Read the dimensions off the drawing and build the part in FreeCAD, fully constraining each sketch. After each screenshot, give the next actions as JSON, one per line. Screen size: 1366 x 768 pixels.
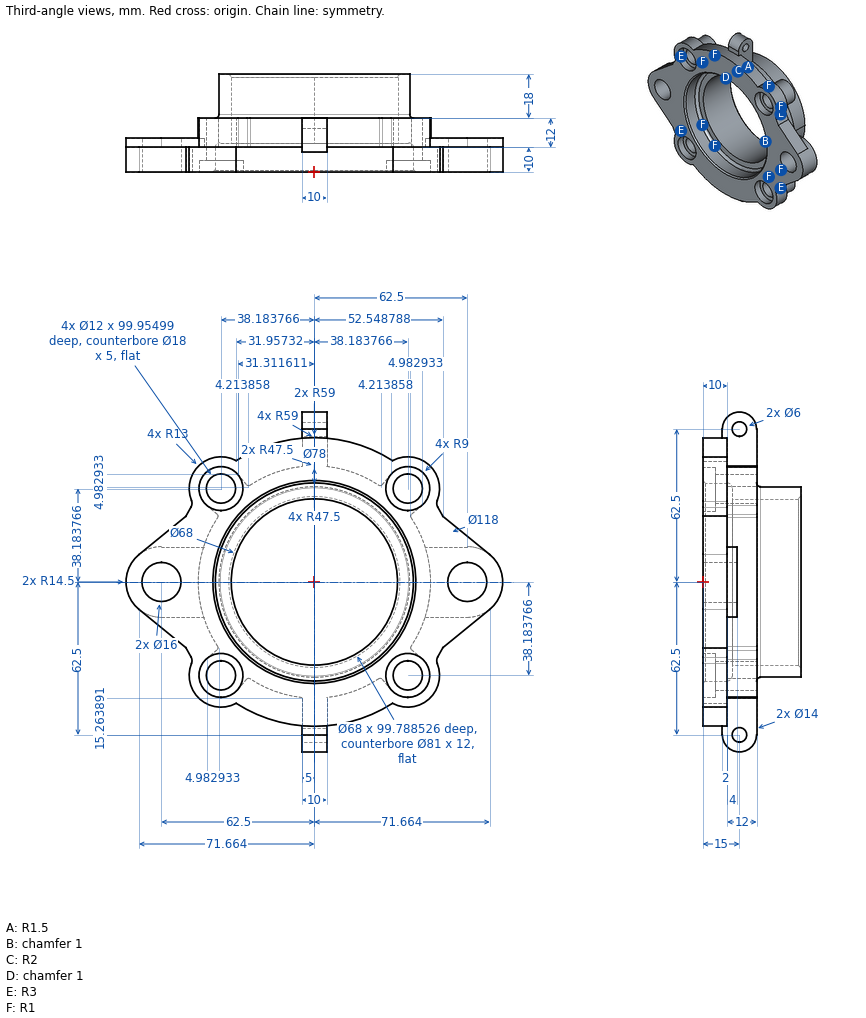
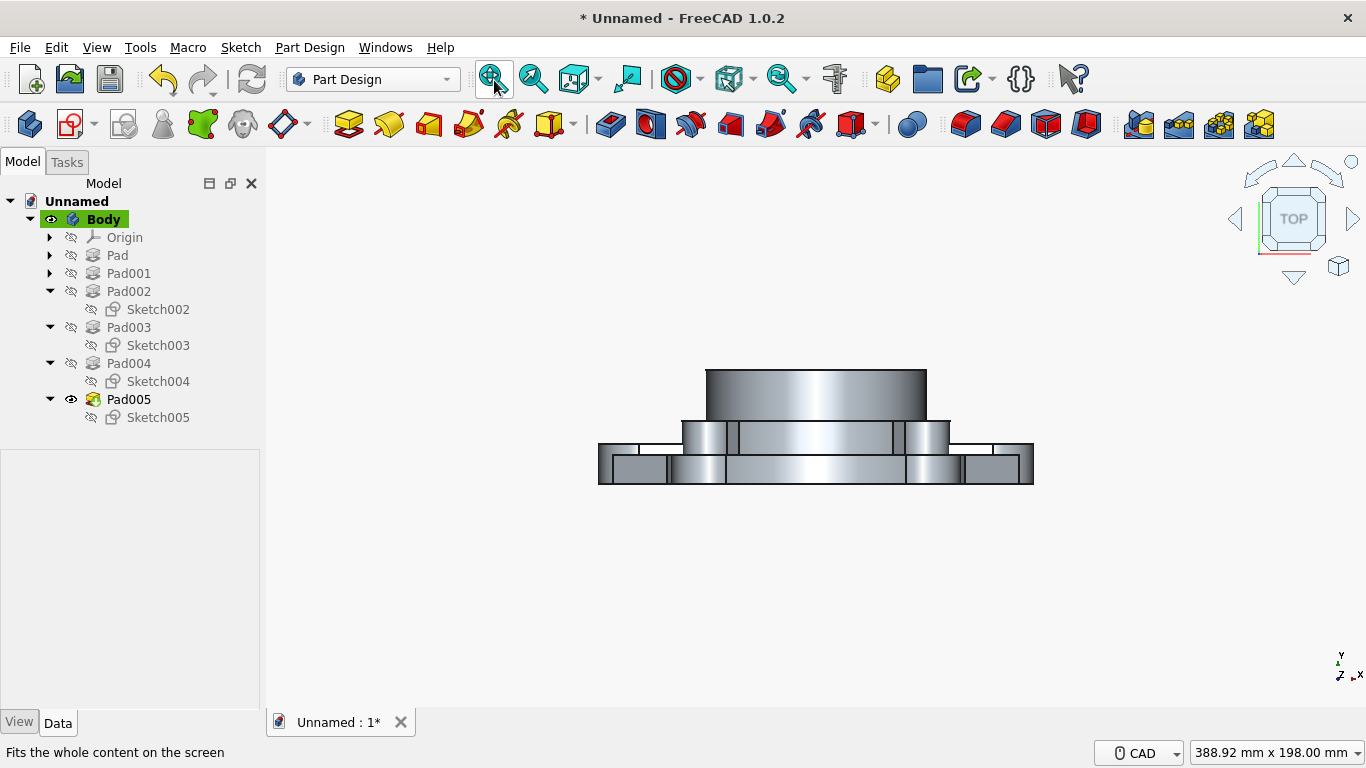
{"action": "left_click", "coordinate": [494, 80]}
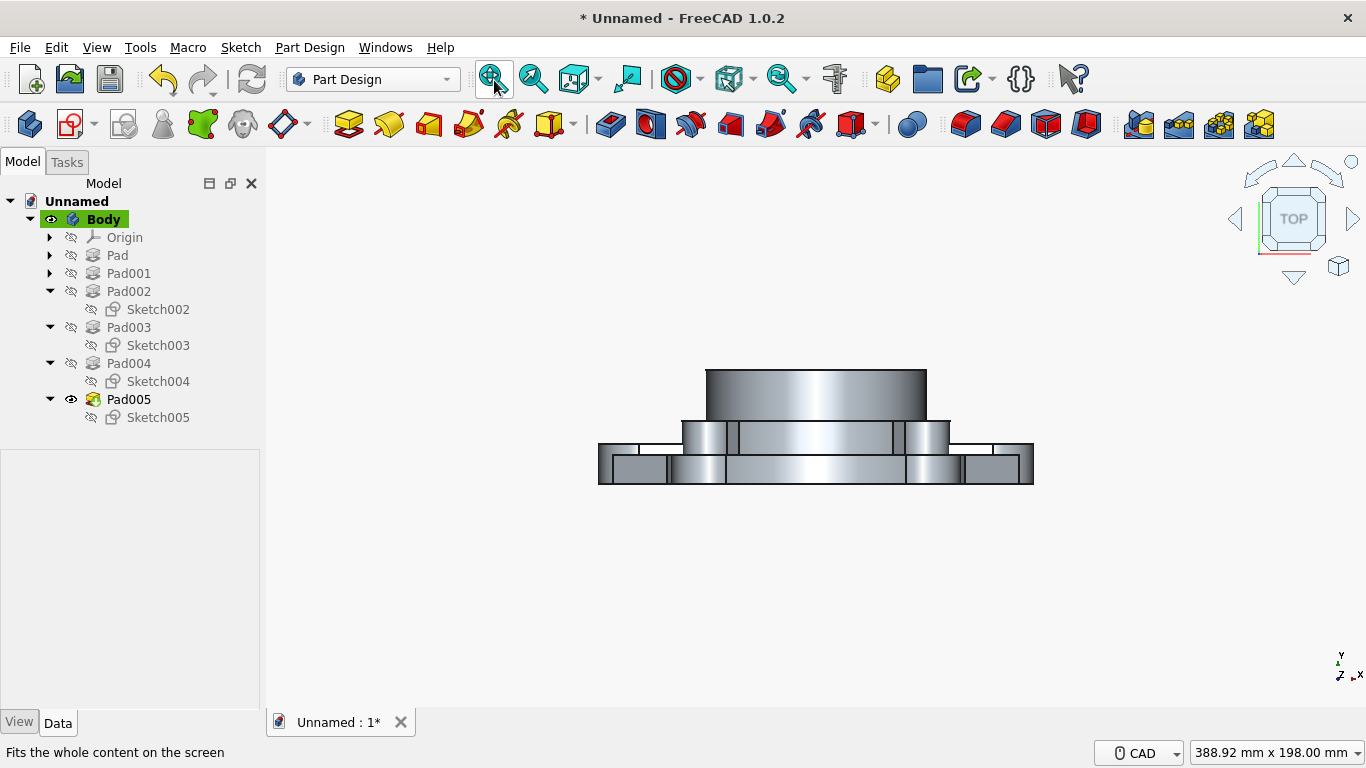
{"action": "key", "text": "1"}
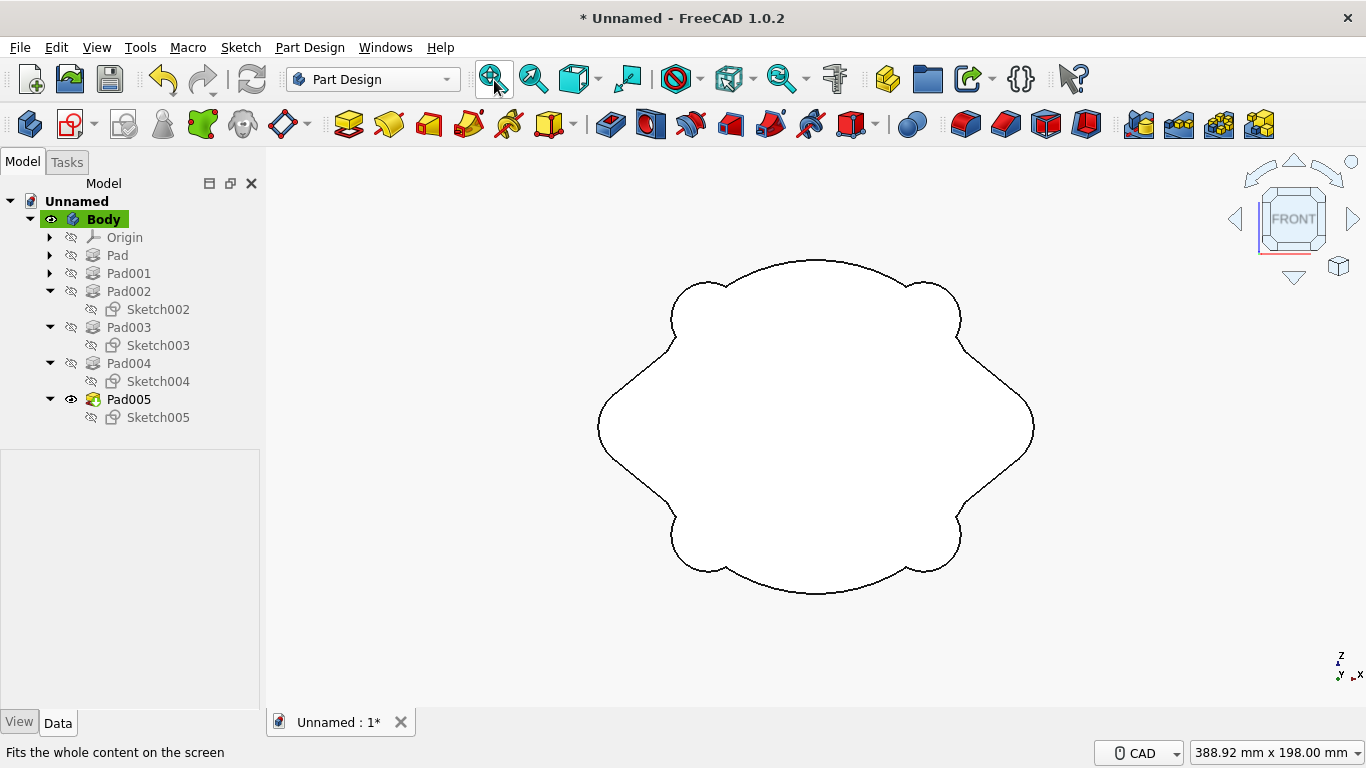
{"action": "key", "text": "3"}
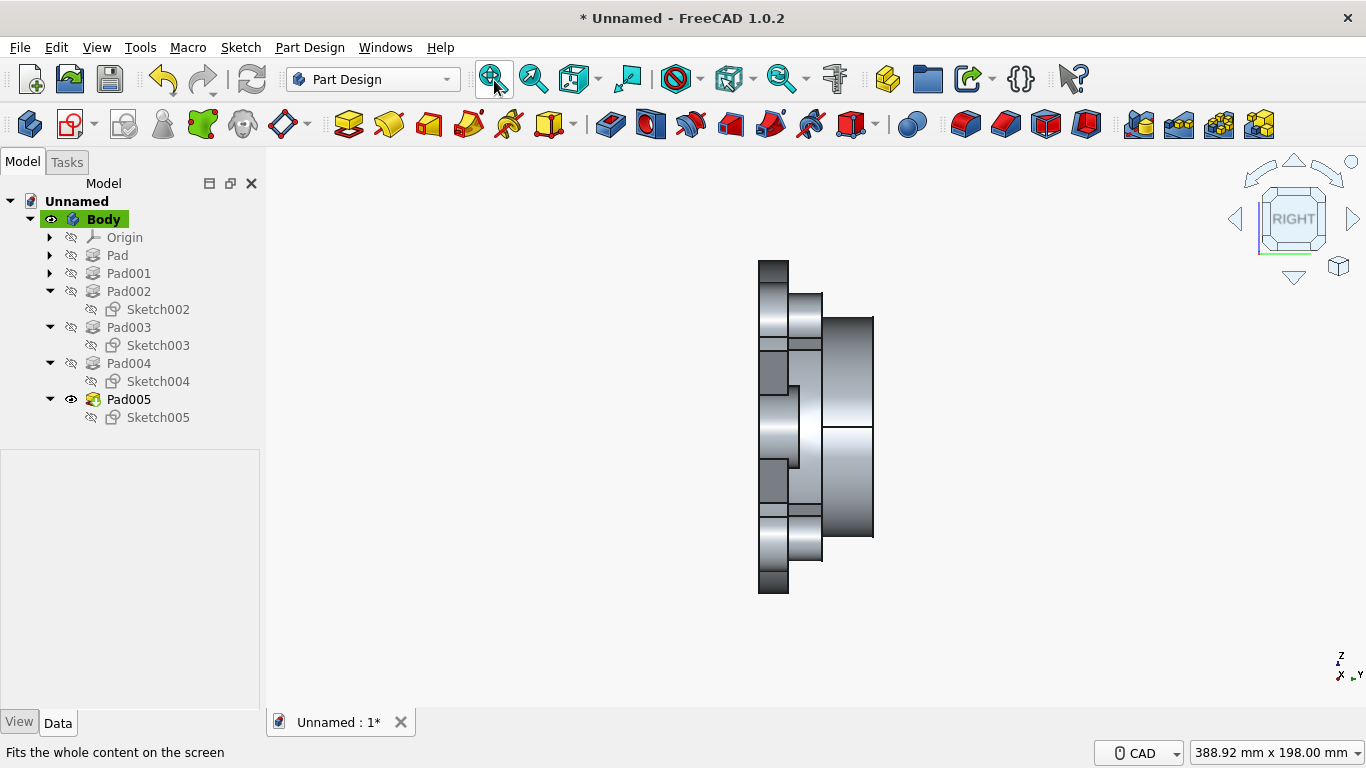
{"action": "key", "text": "5"}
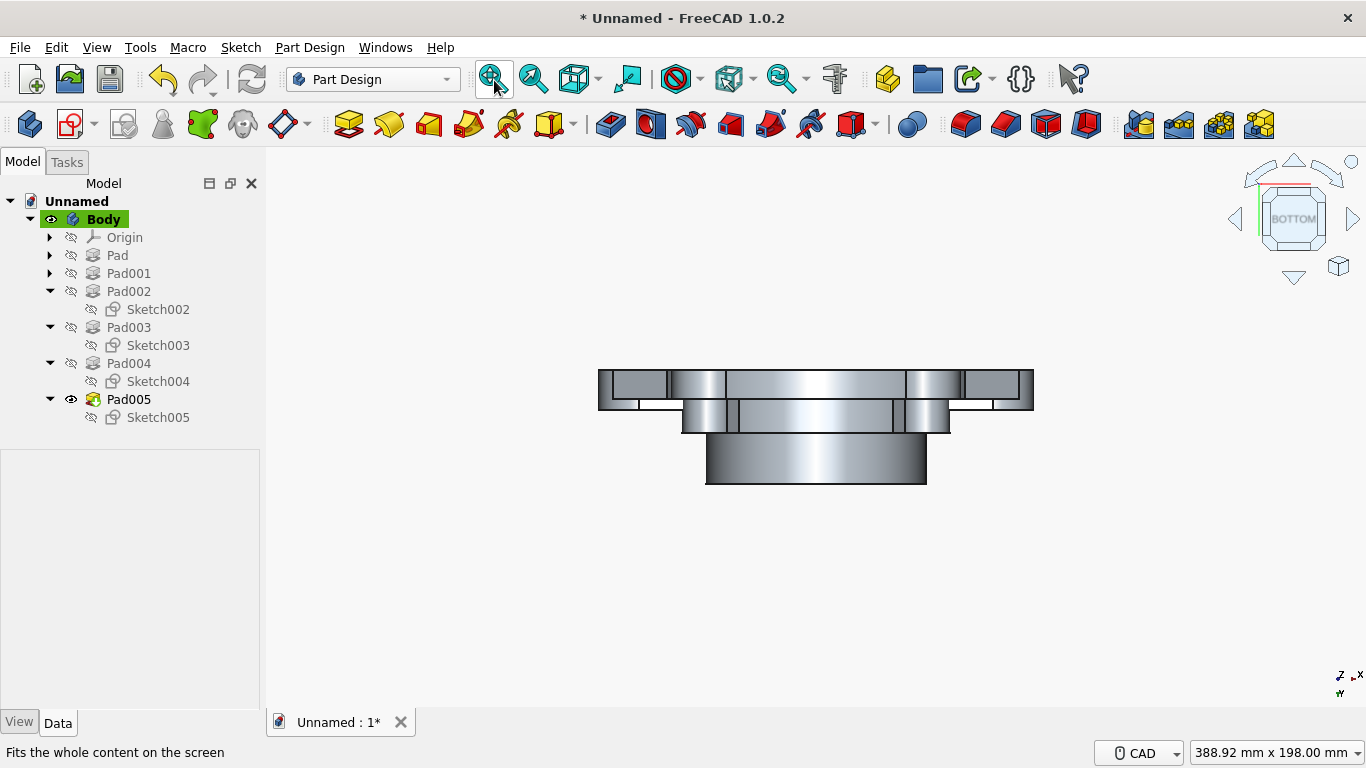
{"action": "left_click", "coordinate": [494, 80]}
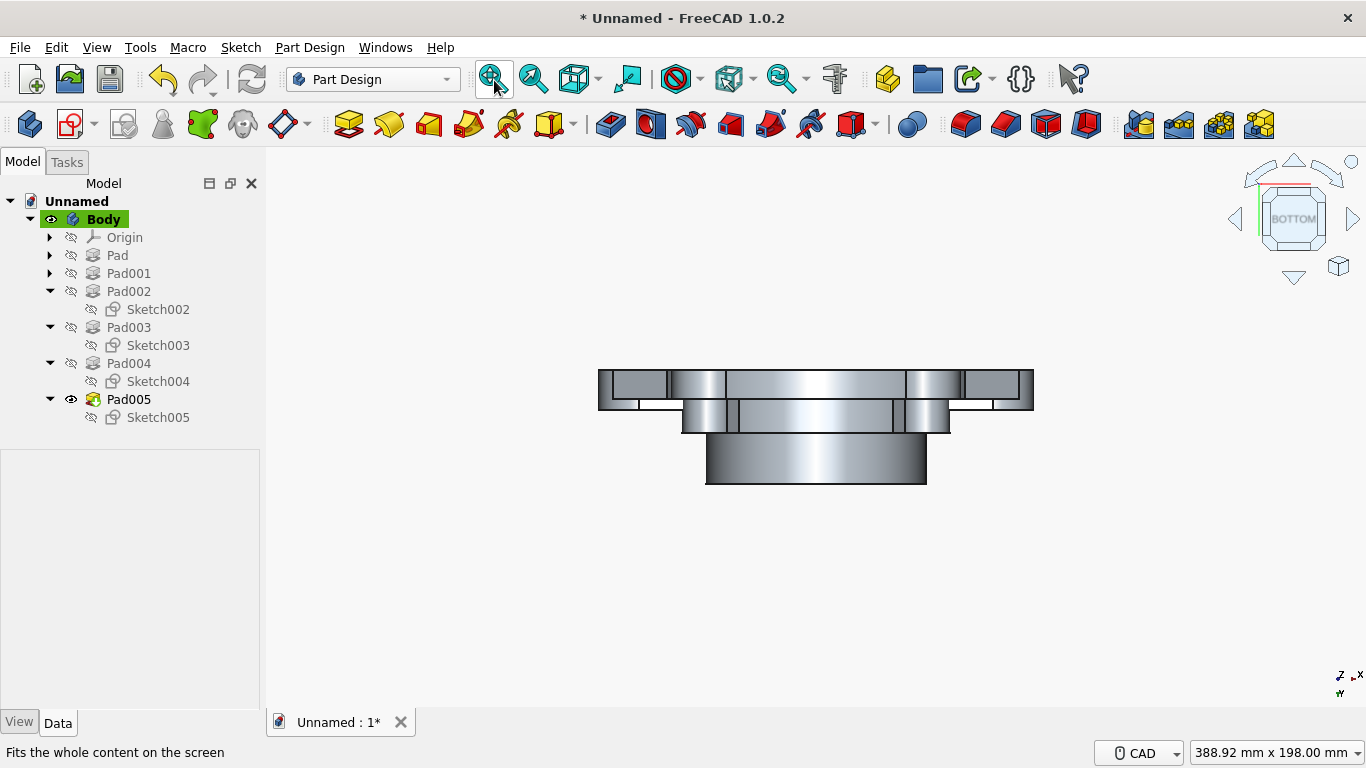
{"action": "key", "text": "4"}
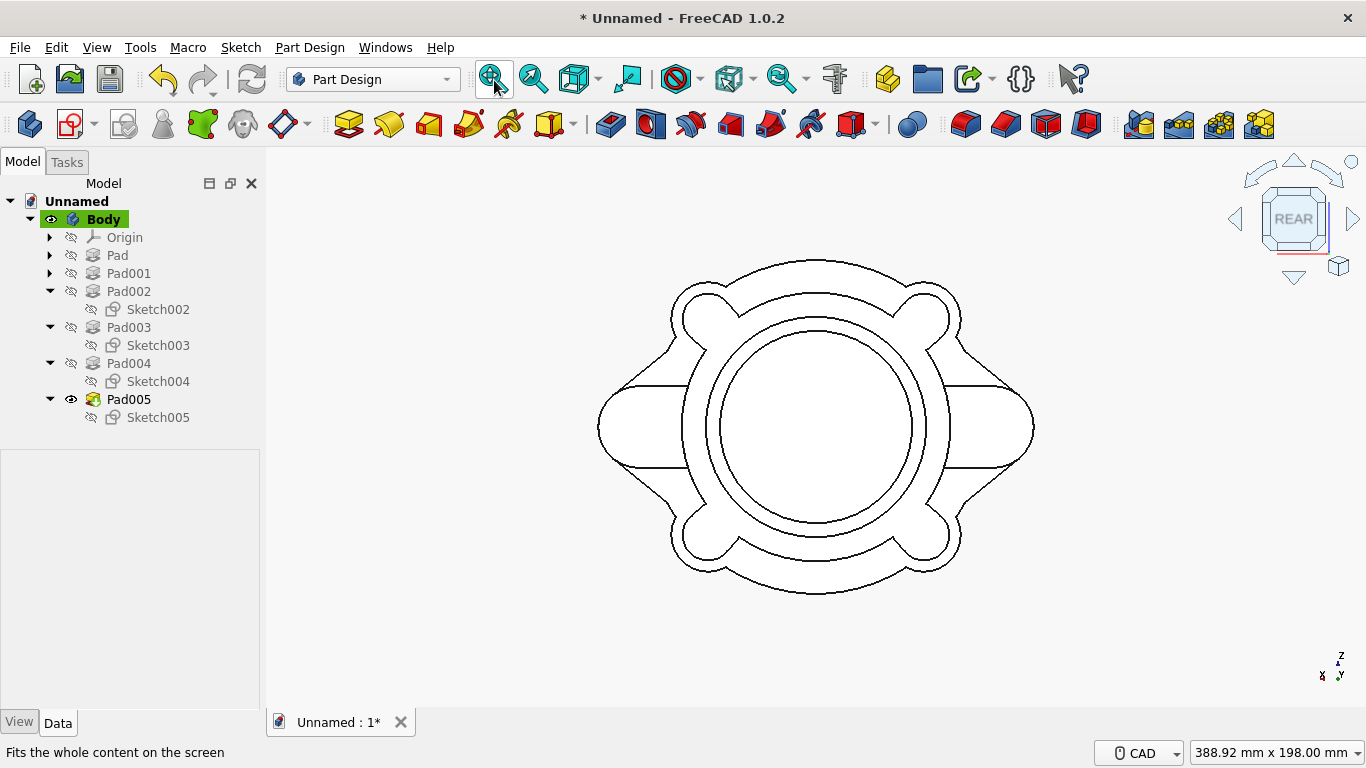
{"action": "key", "text": "6"}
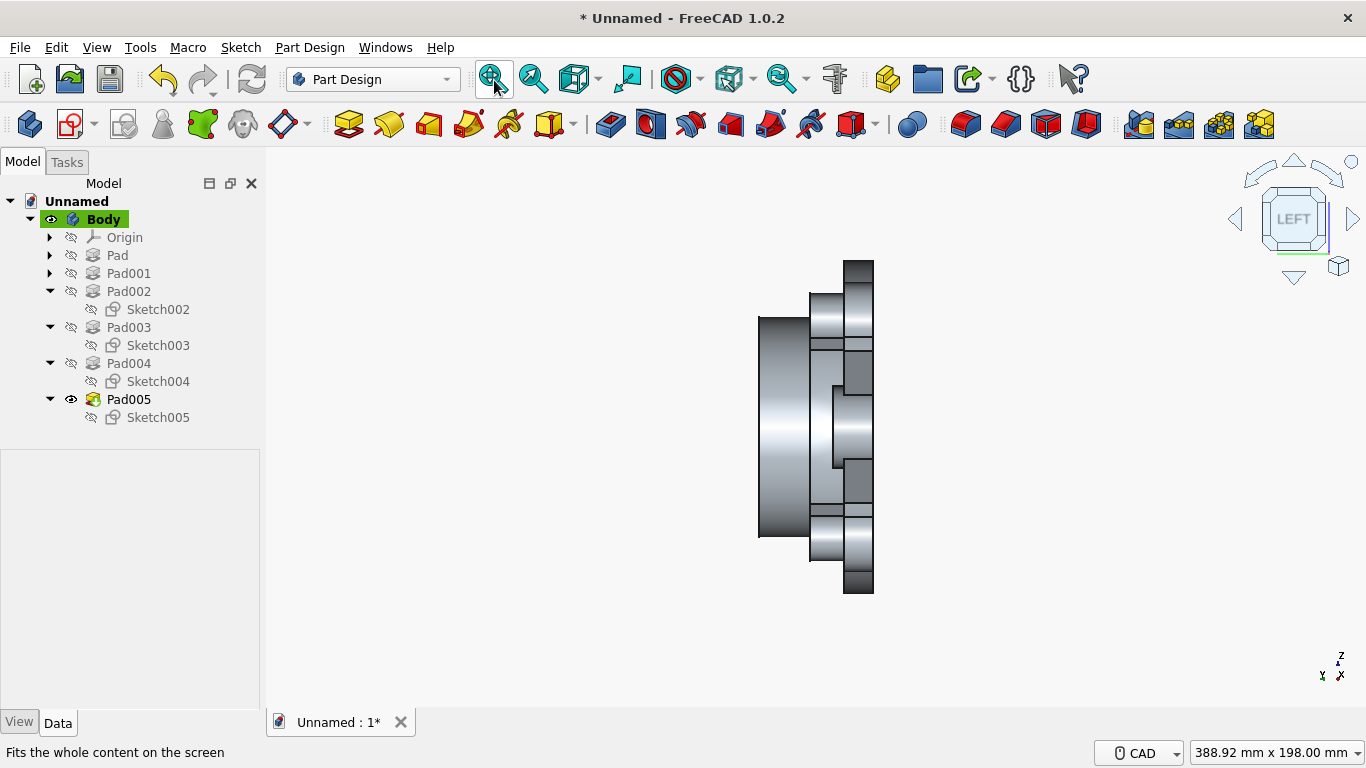
{"action": "key", "text": "v 3"}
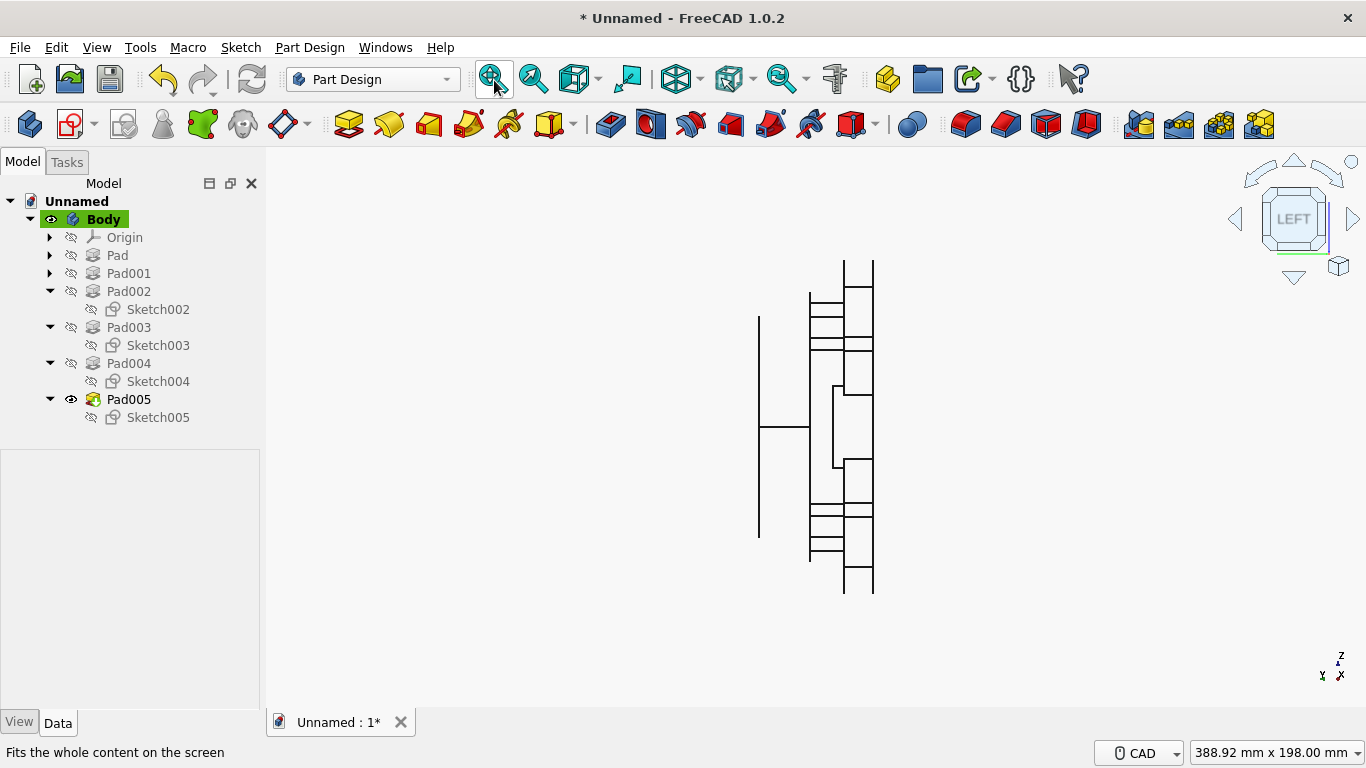
{"action": "key", "text": "0"}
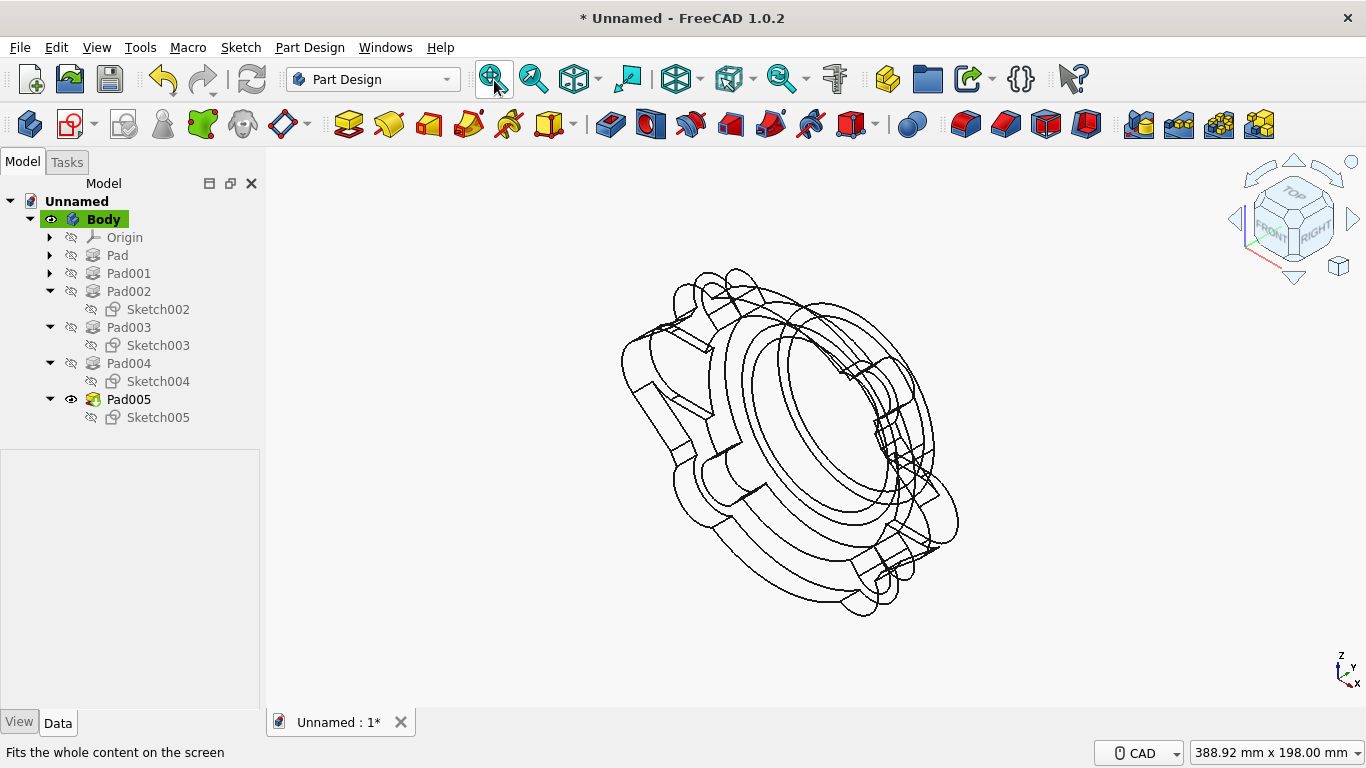
{"action": "left_click", "coordinate": [742, 379]}